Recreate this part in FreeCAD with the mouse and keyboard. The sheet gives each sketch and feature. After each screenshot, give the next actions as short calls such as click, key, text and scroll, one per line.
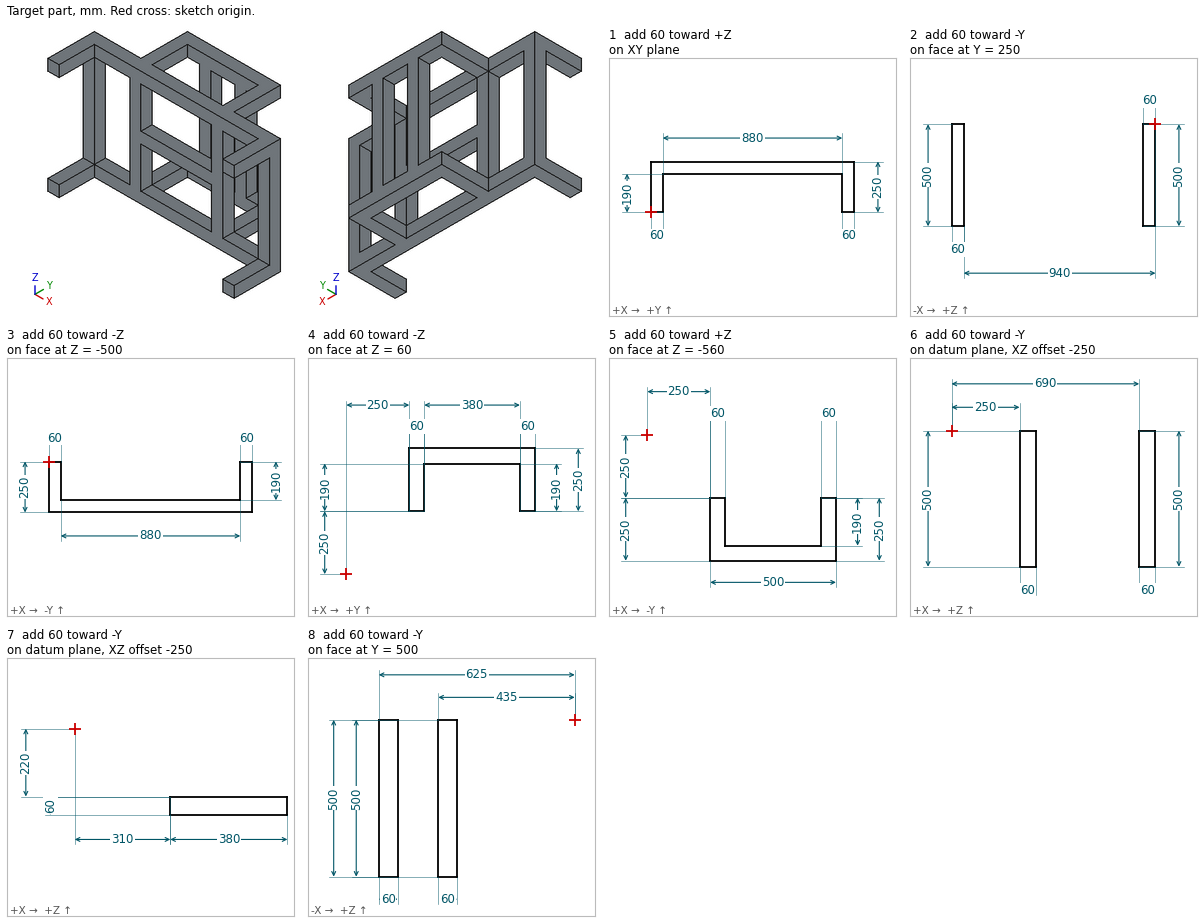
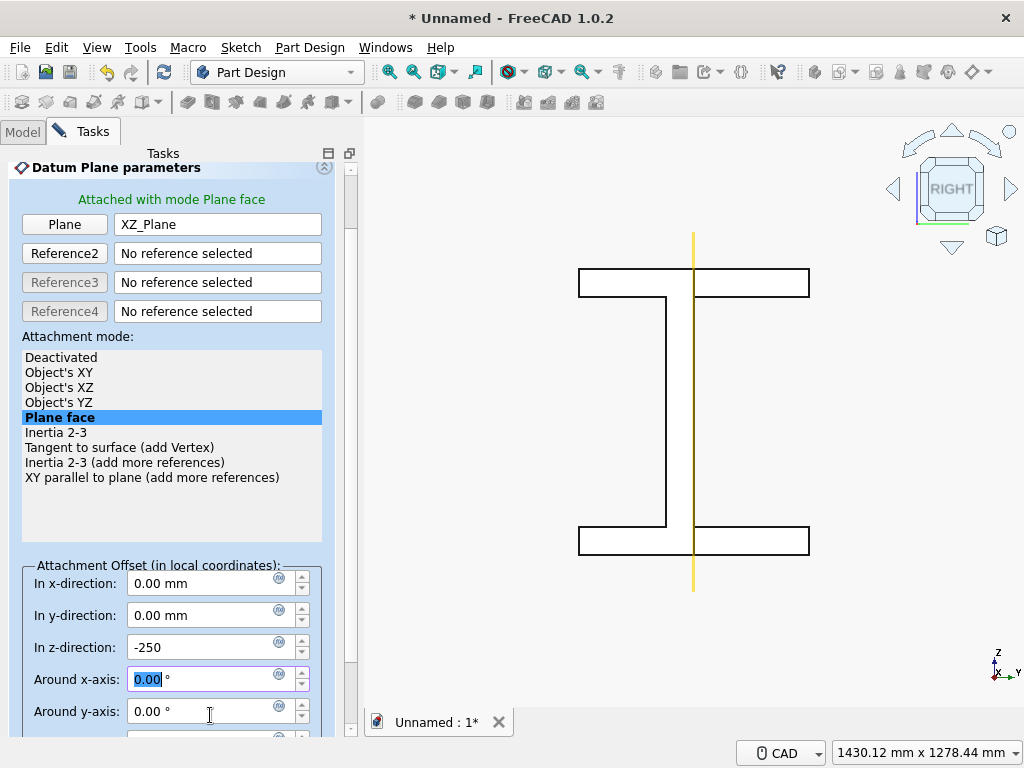
scroll(351, 450, up, 2)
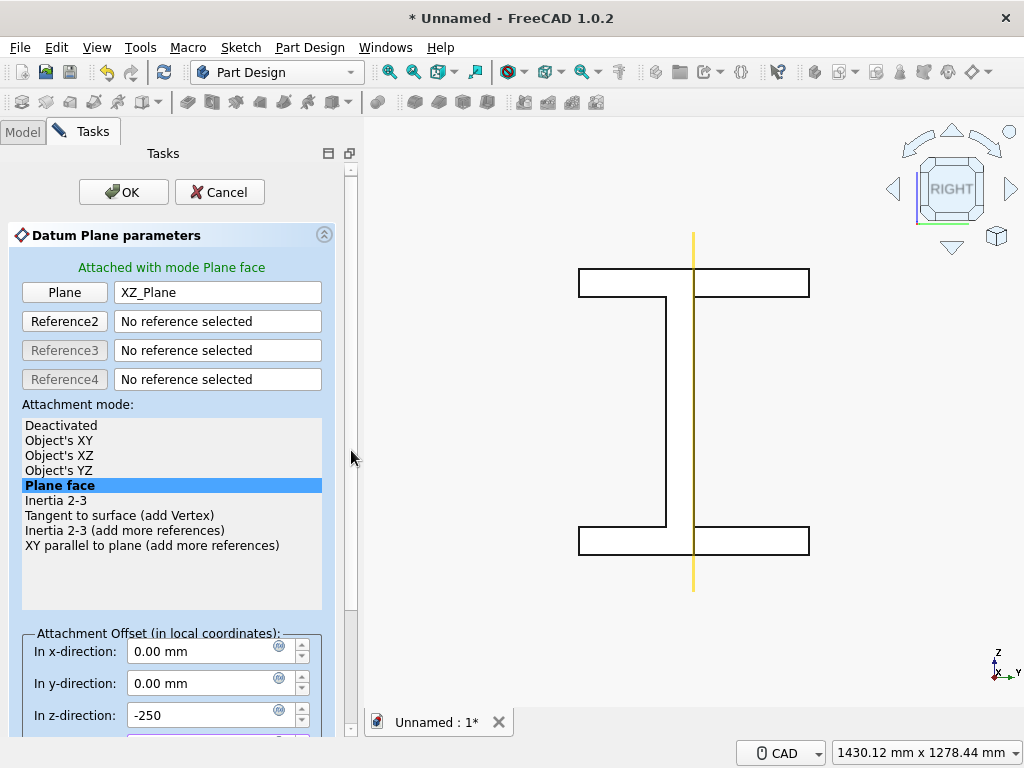
click(124, 192)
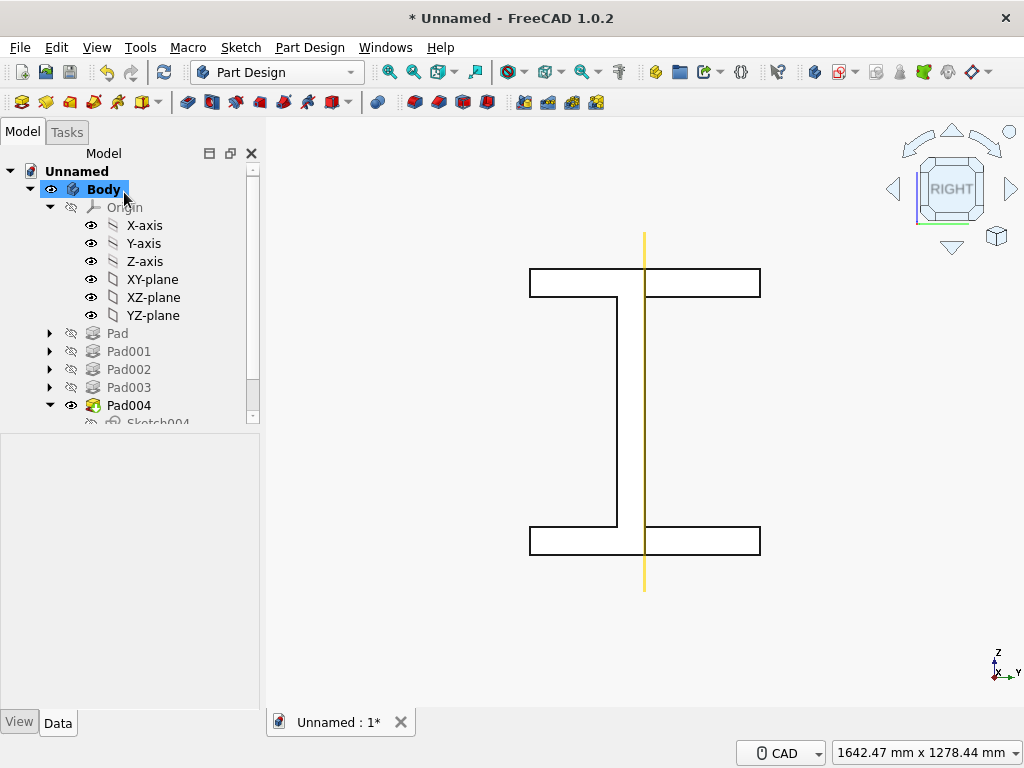
scroll(100, 293, down, 3)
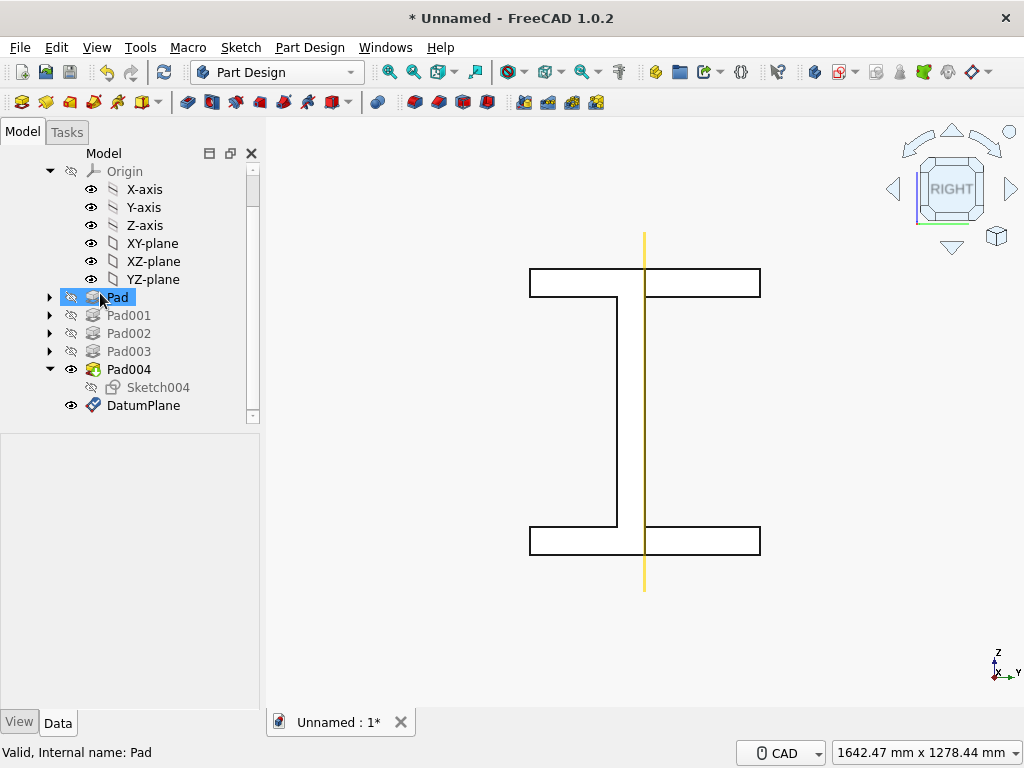
click(116, 405)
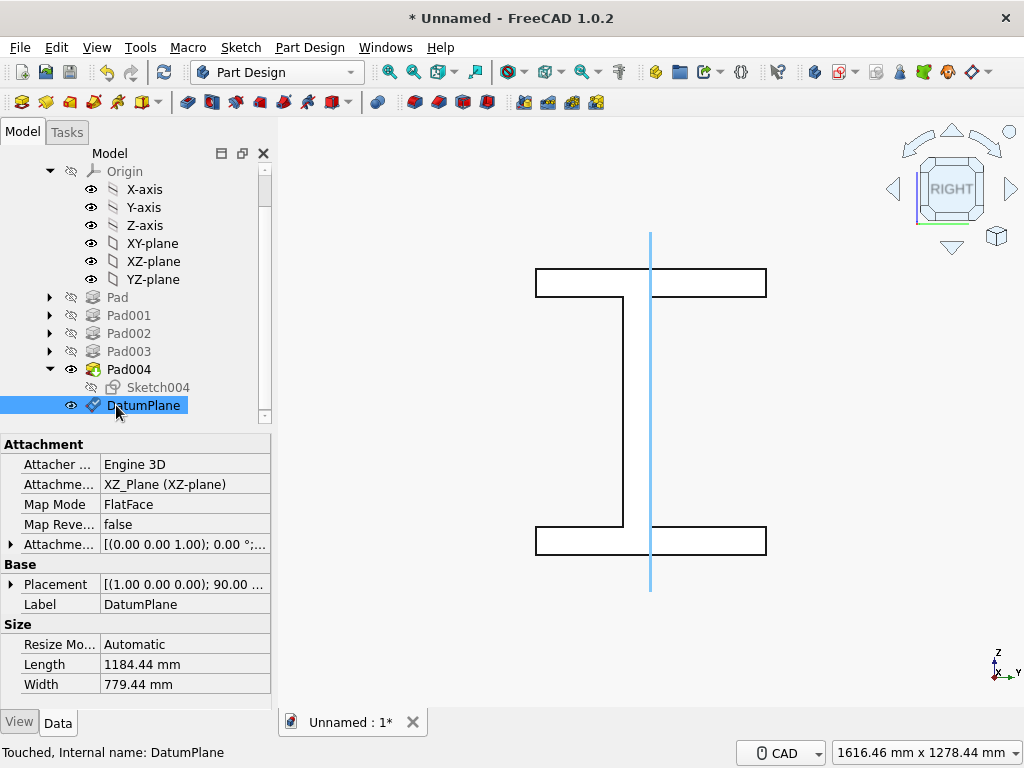
click(840, 72)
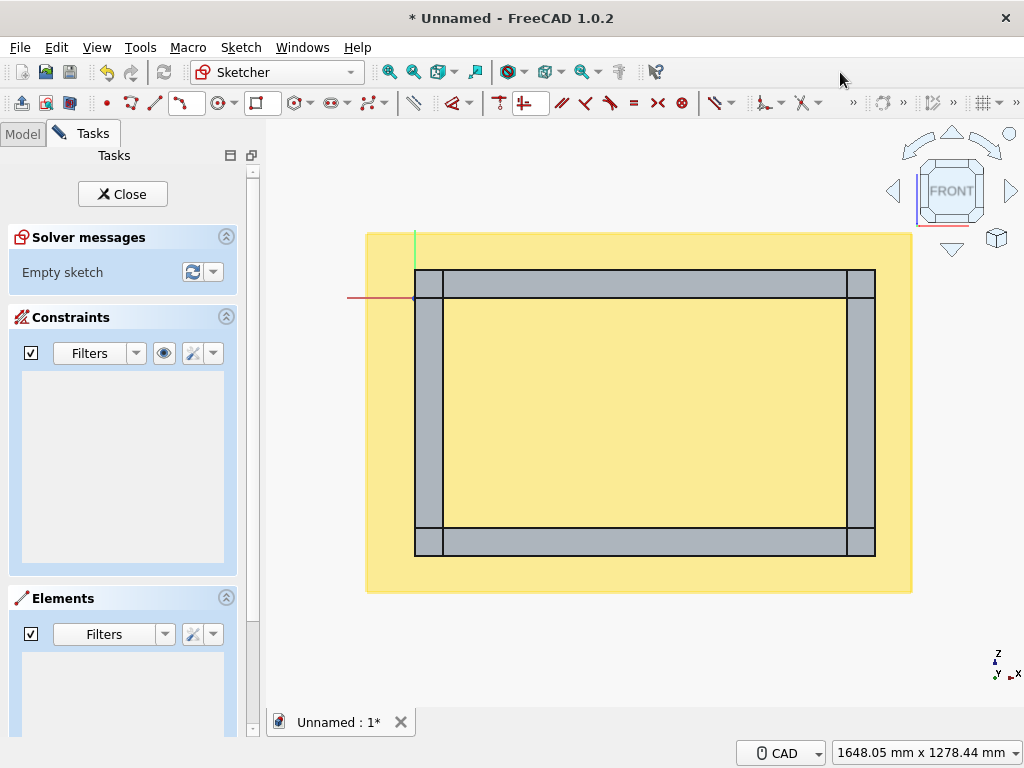
click(70, 104)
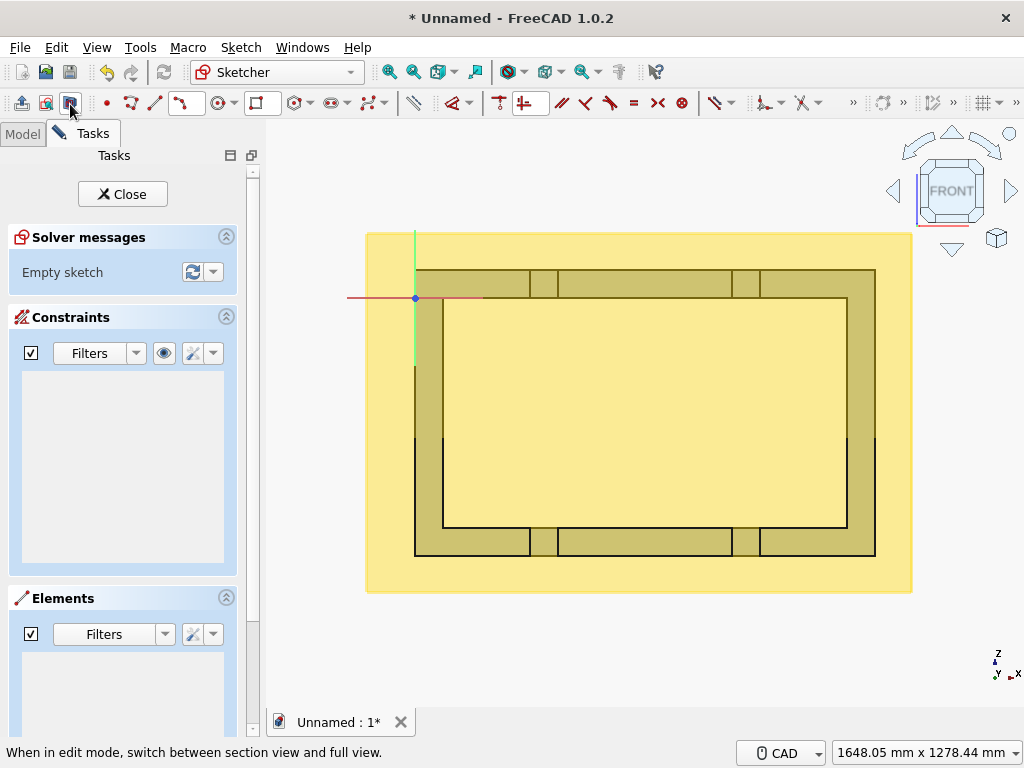
click(256, 104)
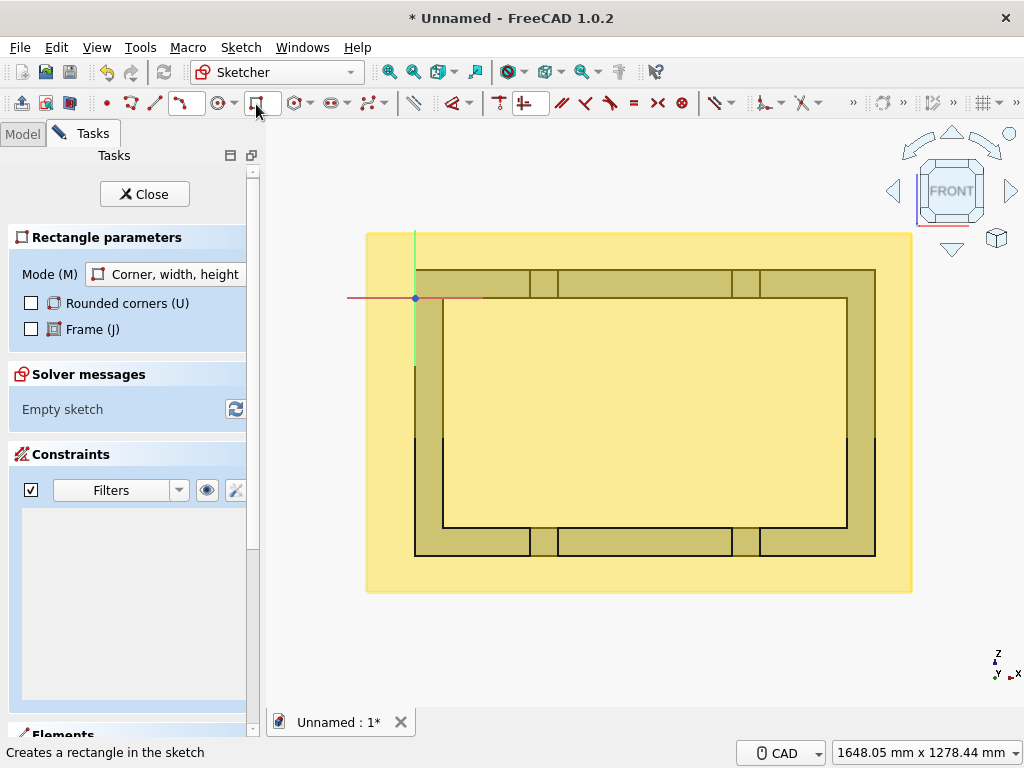
click(530, 298)
click(558, 528)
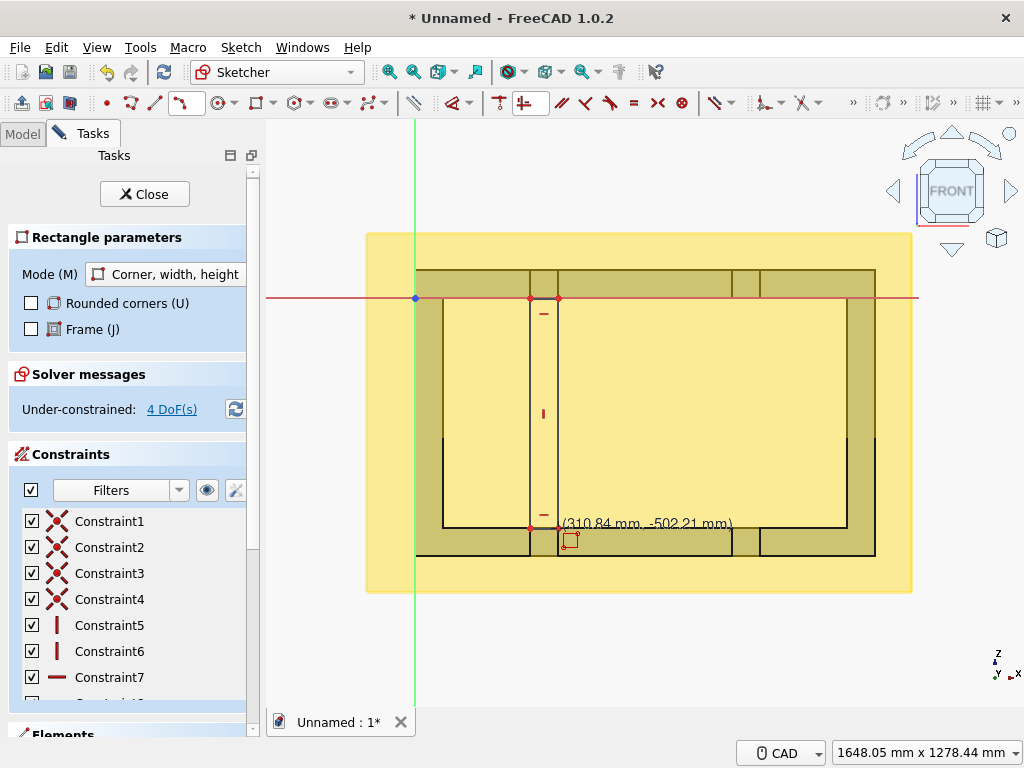
click(732, 298)
click(760, 528)
key(Escape)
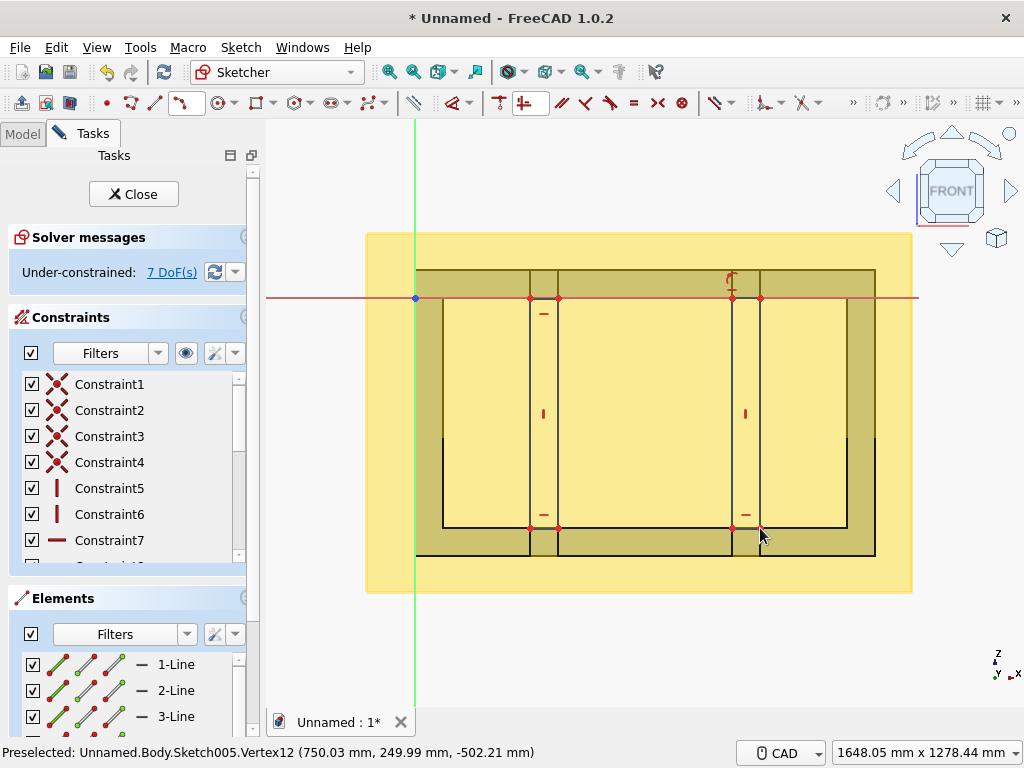
click(530, 299)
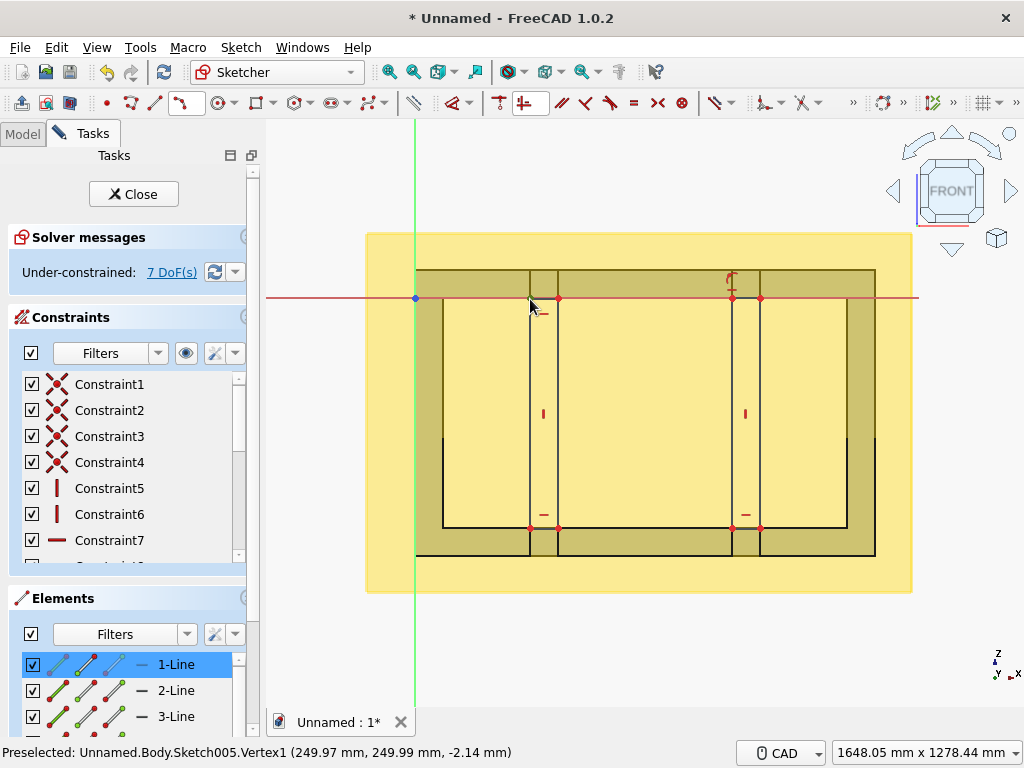
click(334, 298)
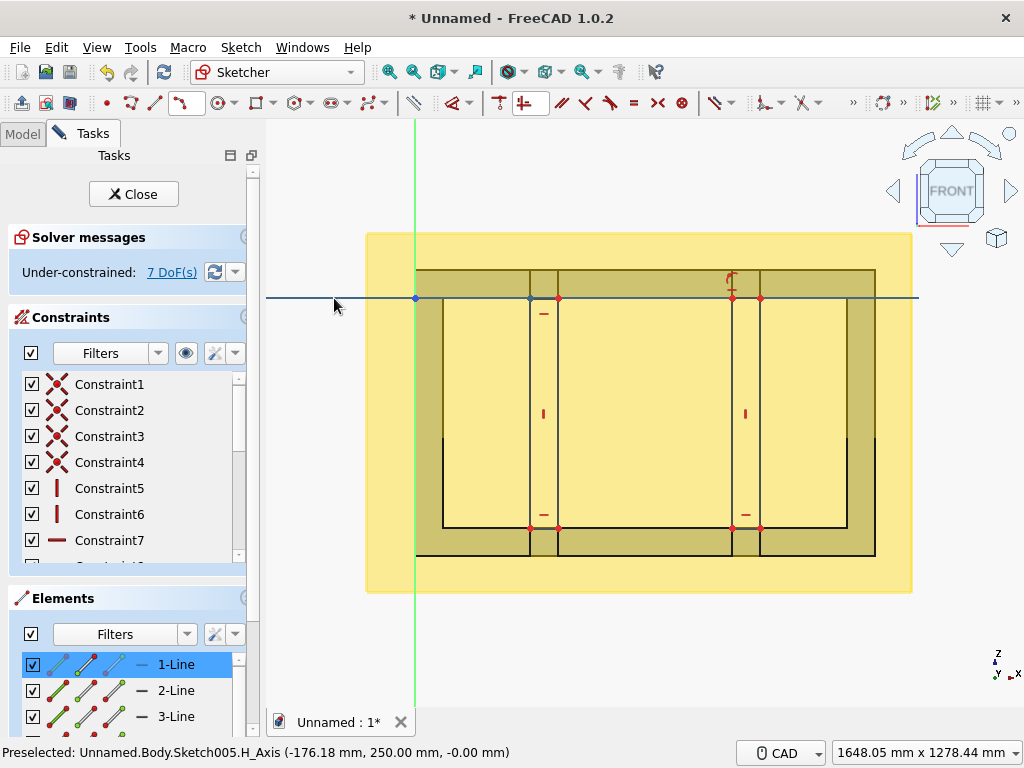
click(500, 104)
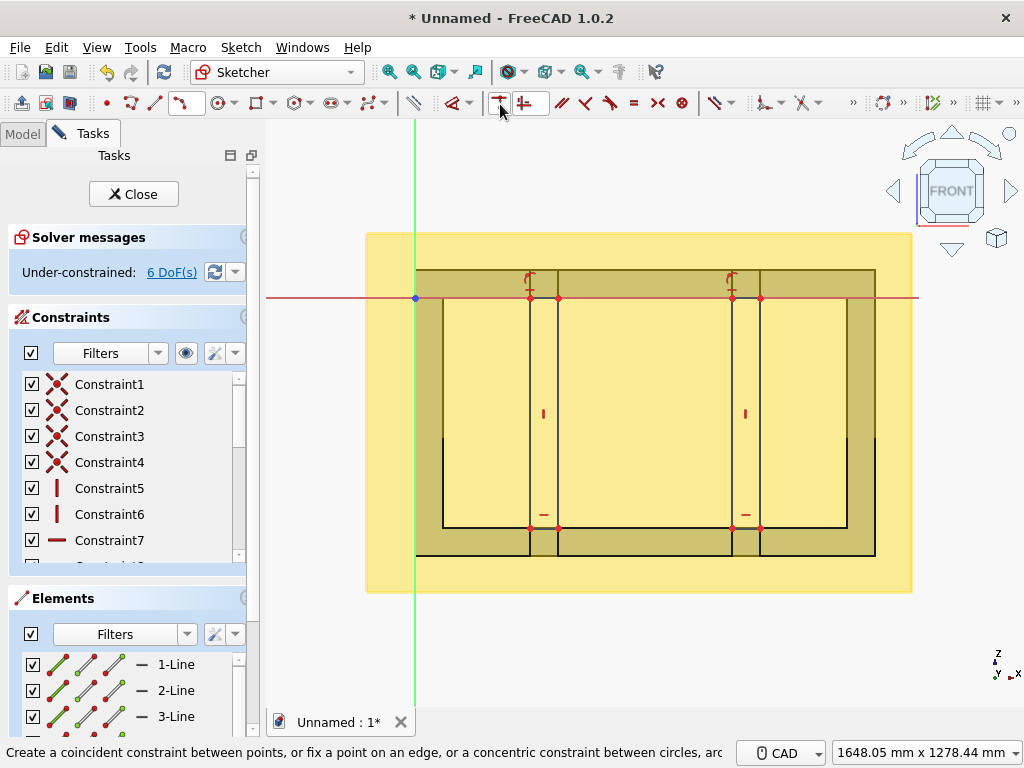
click(452, 104)